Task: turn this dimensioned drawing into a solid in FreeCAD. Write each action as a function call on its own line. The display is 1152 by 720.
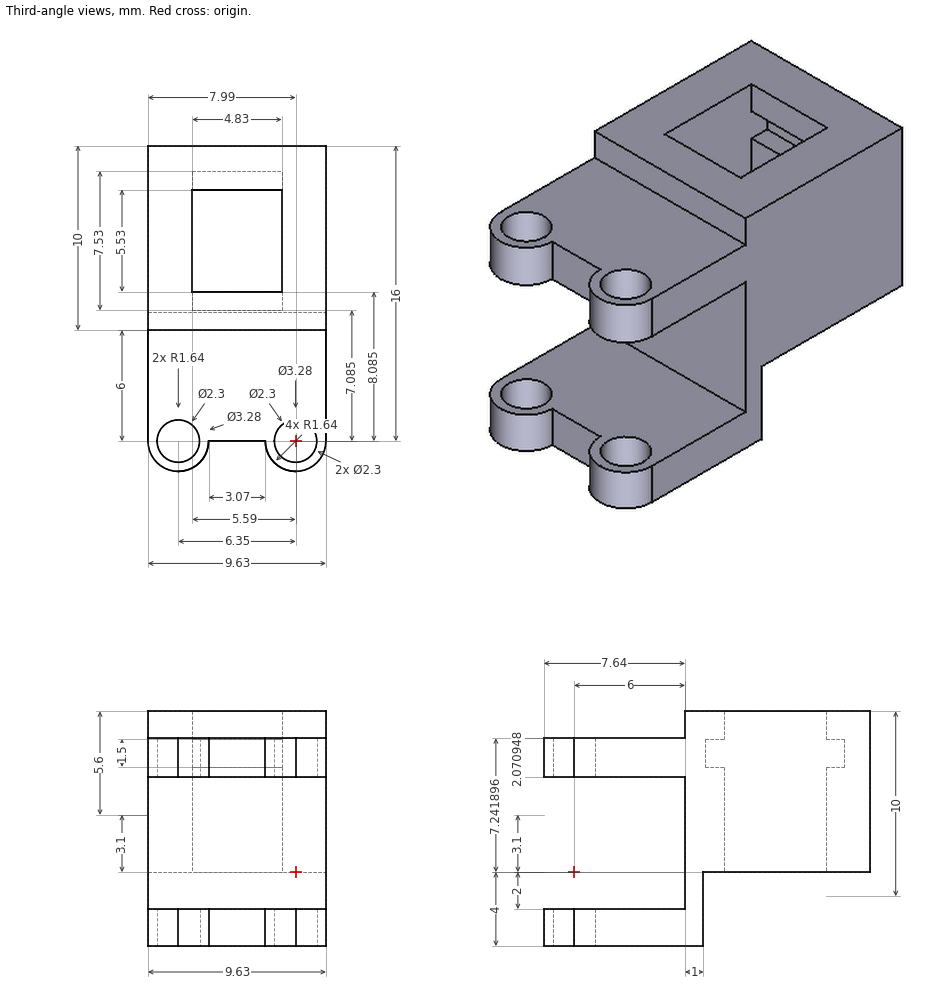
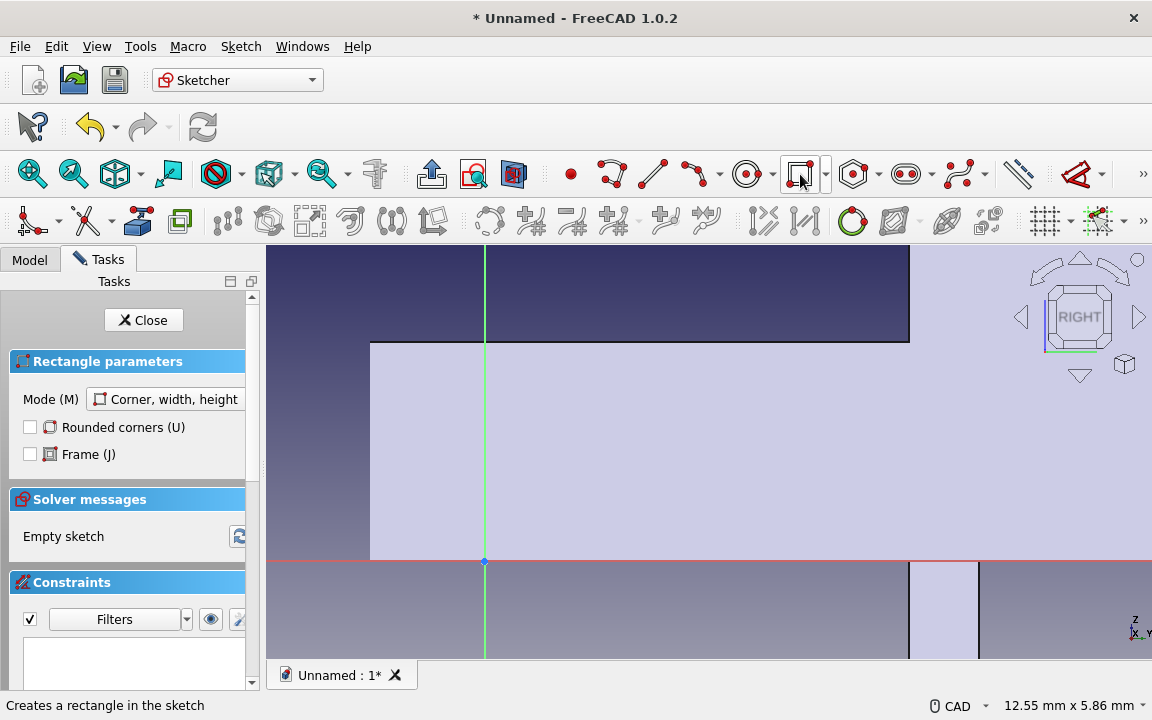
click(369, 342)
click(909, 561)
key(Escape)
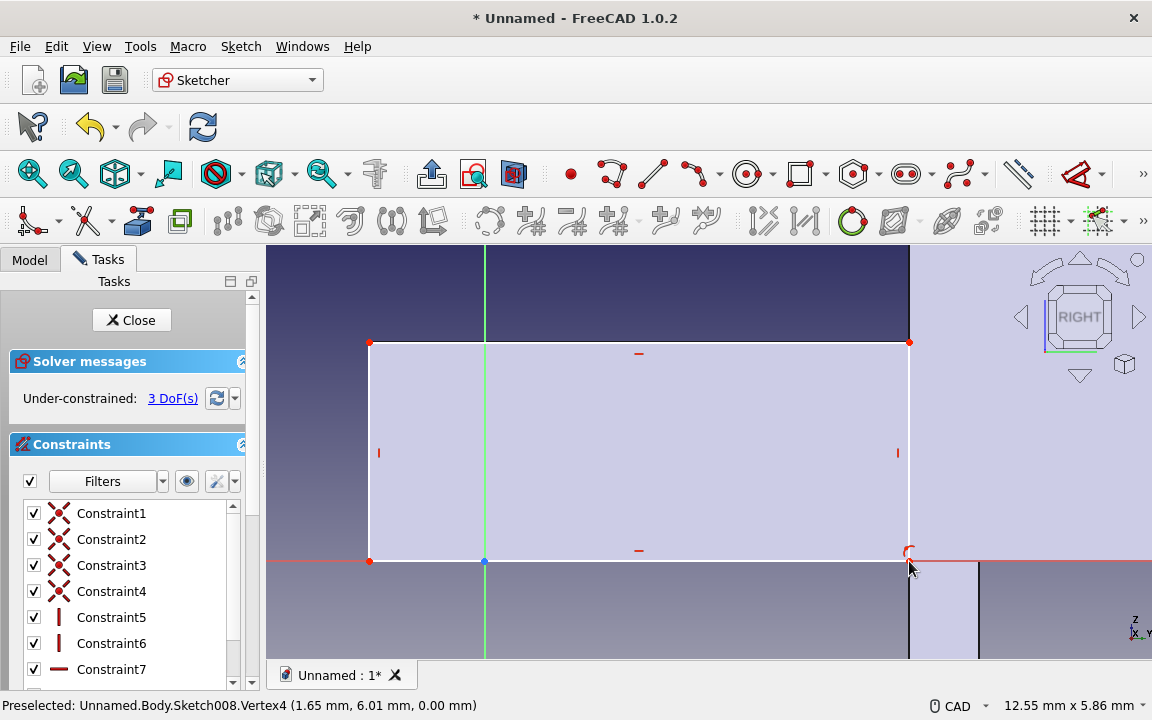
click(1076, 174)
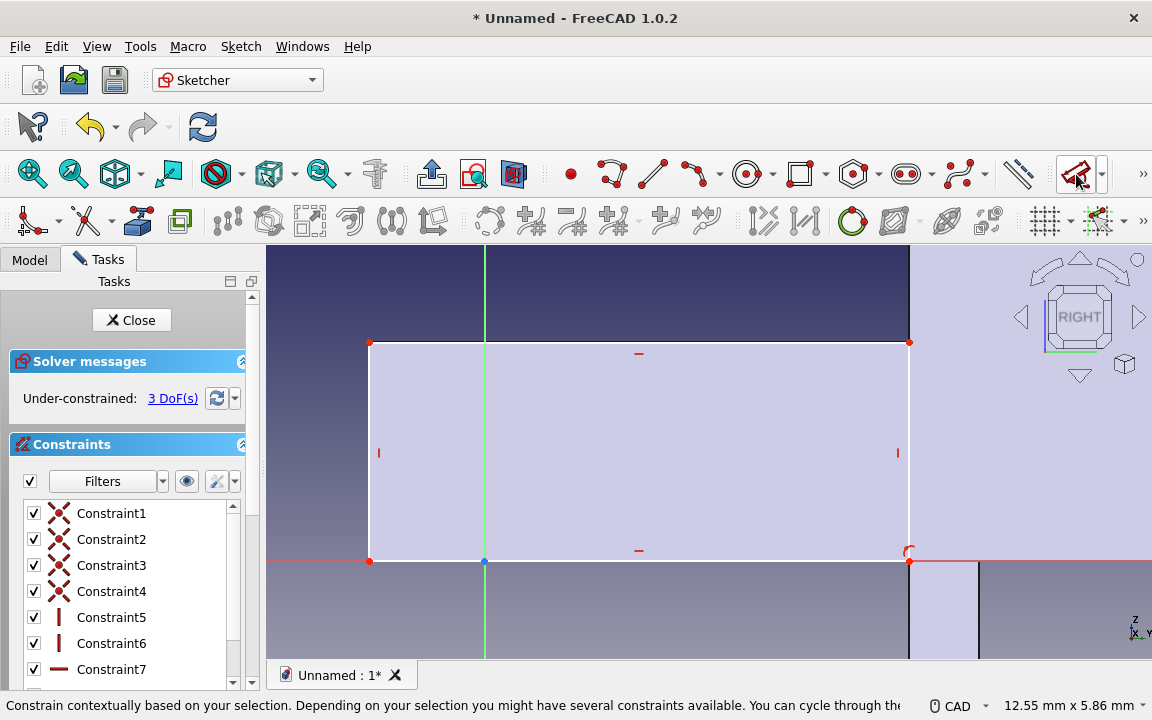
click(909, 561)
click(697, 595)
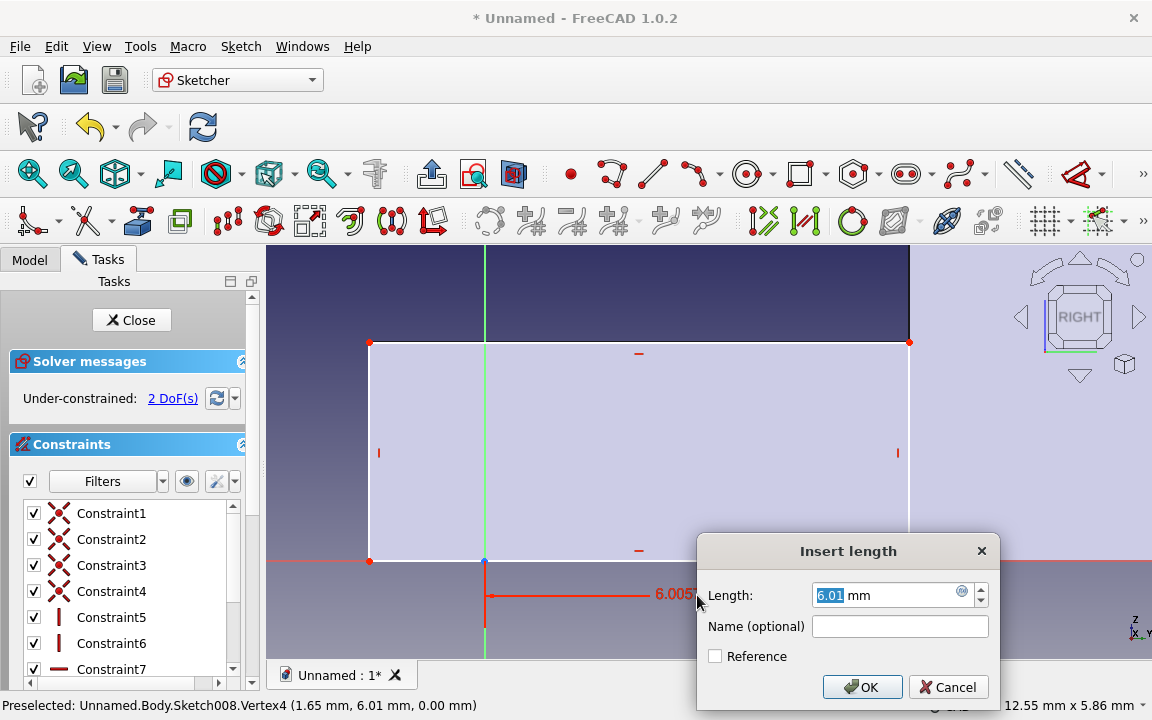
text(6)
key(Return)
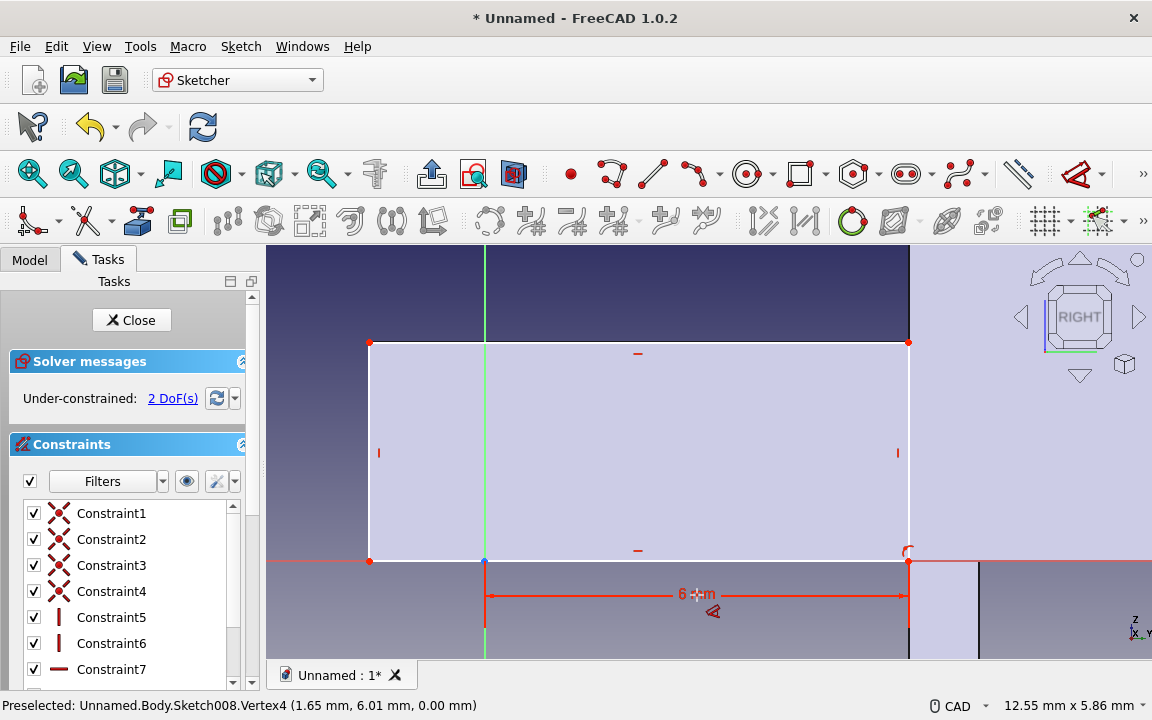
click(369, 408)
click(335, 452)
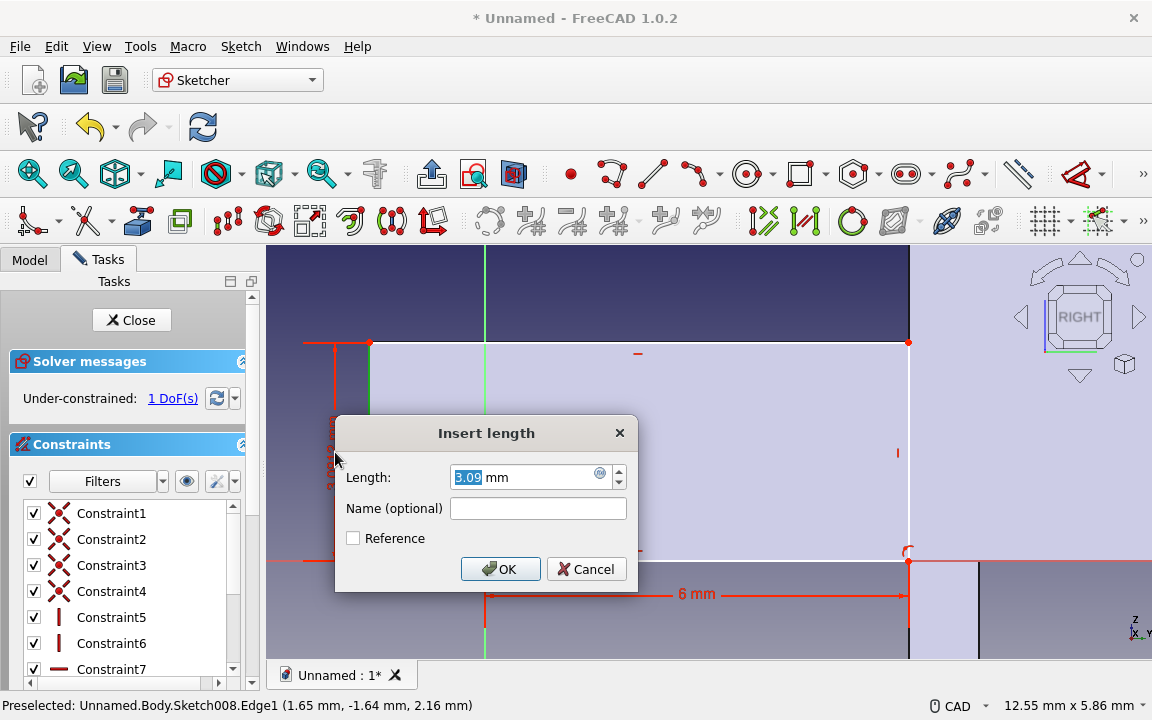
text(3.1)
key(Return)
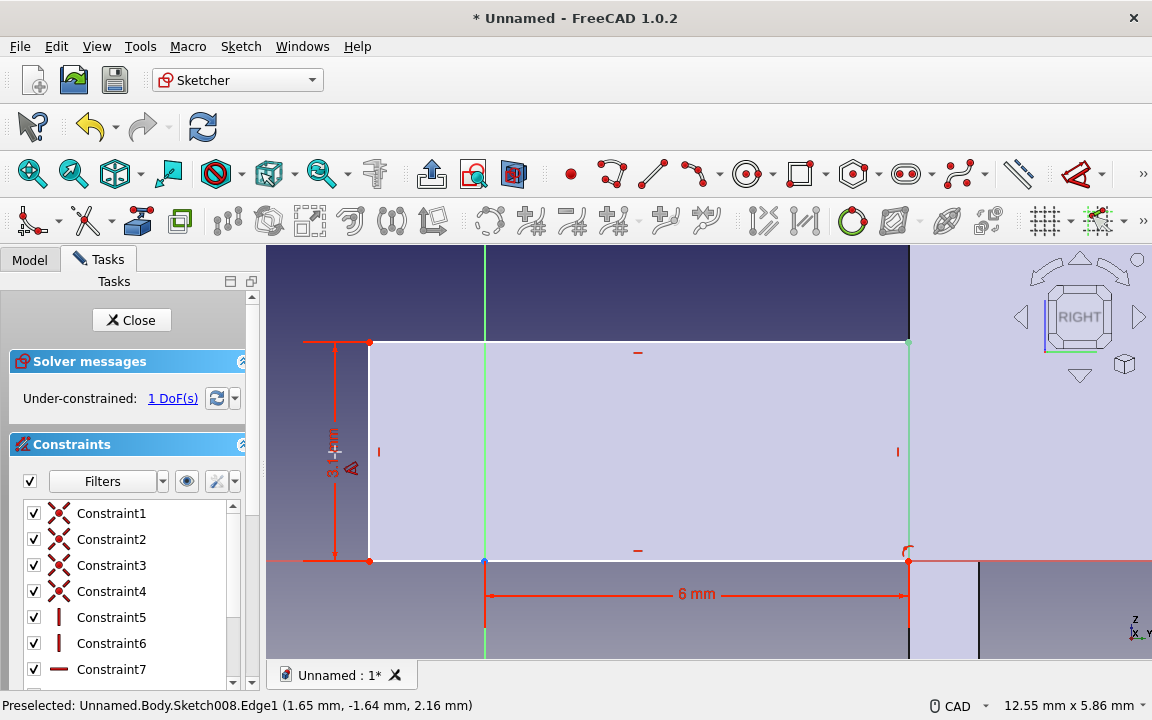
click(531, 561)
click(515, 595)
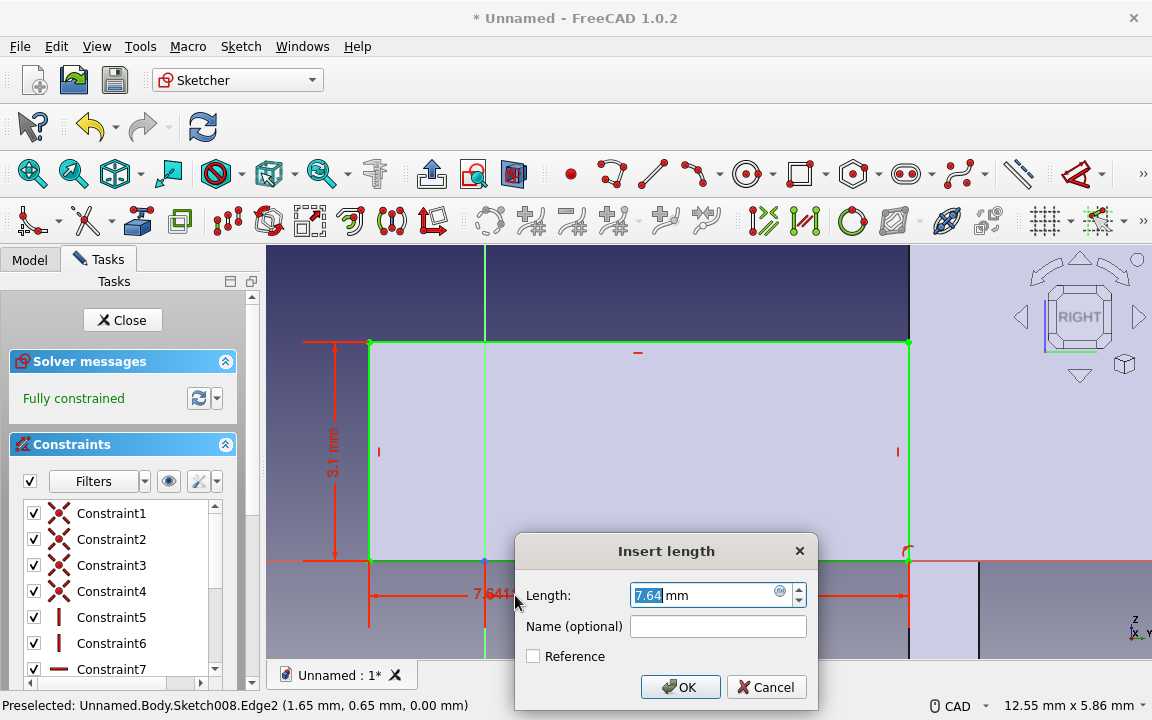
text(7.64)
key(Return)
key(Escape)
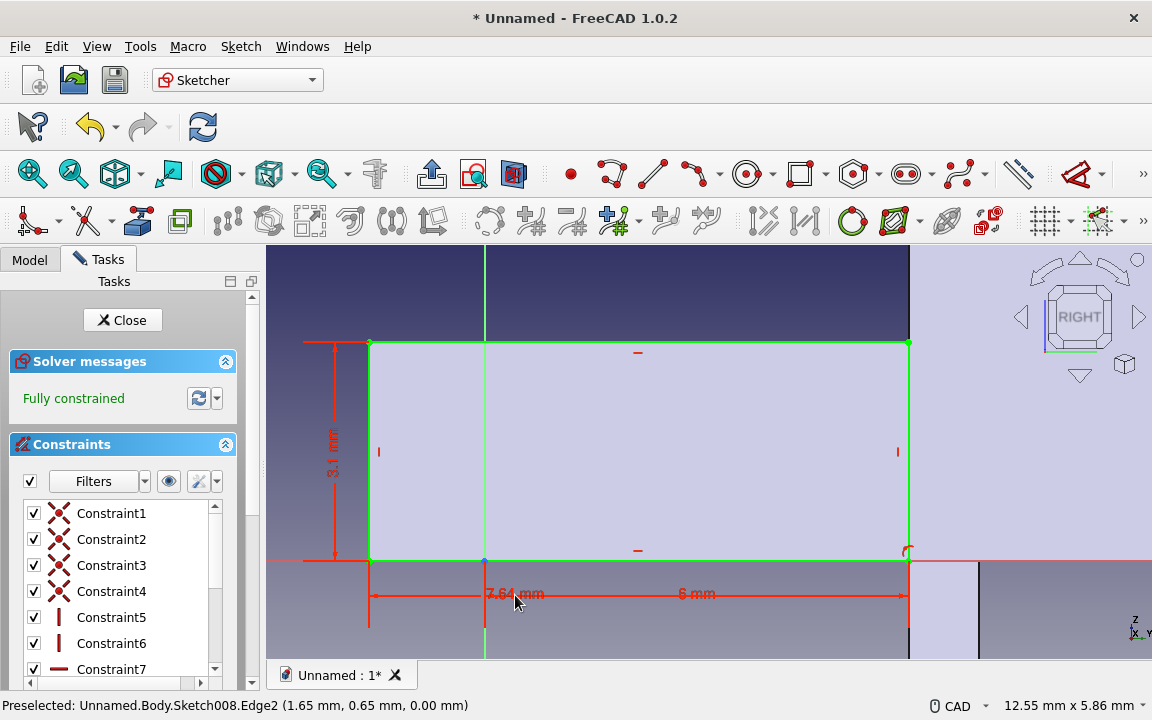
click(123, 320)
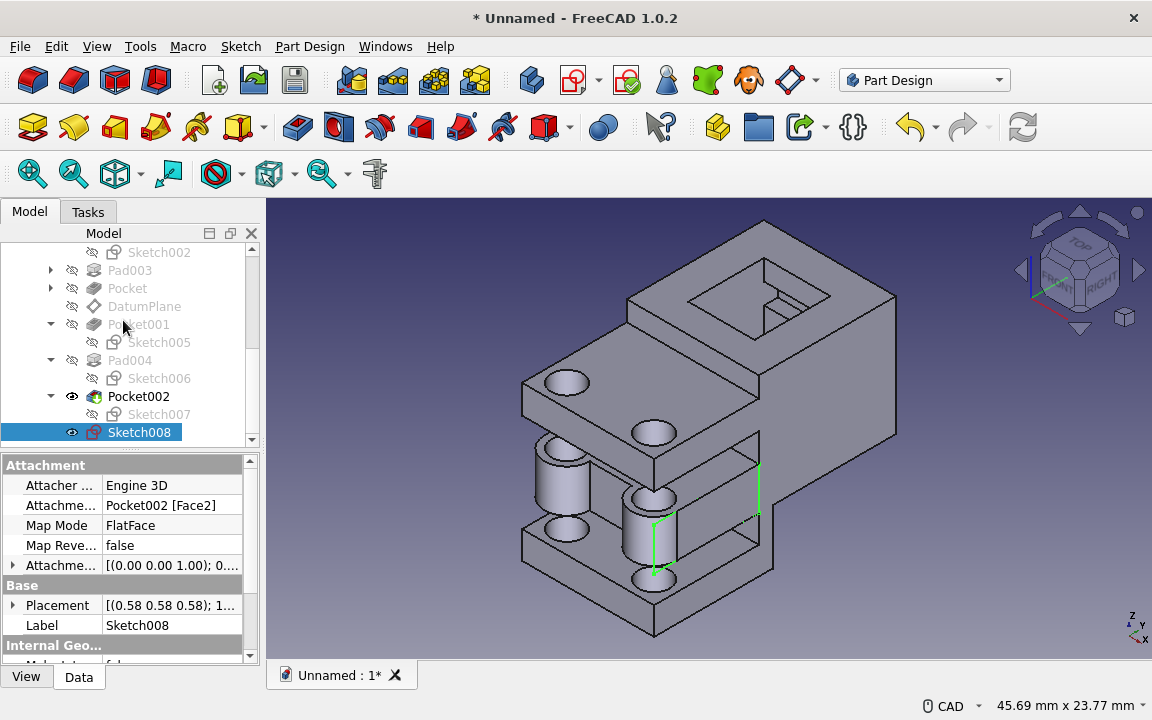
click(298, 128)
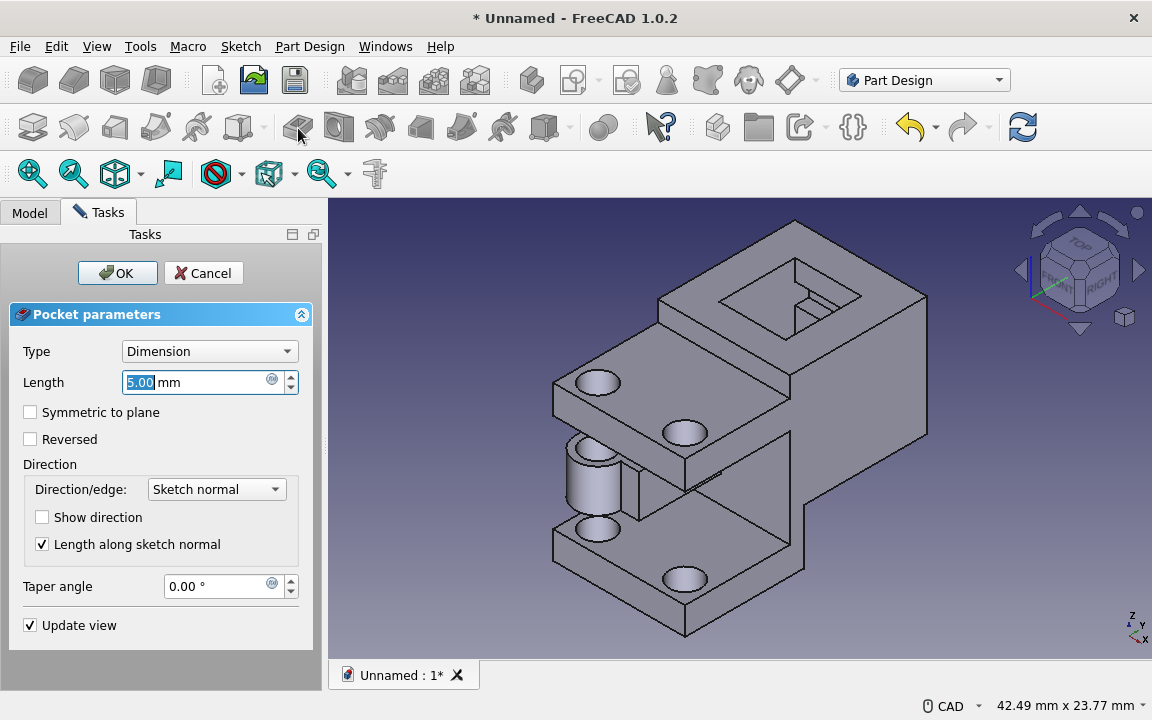
click(210, 352)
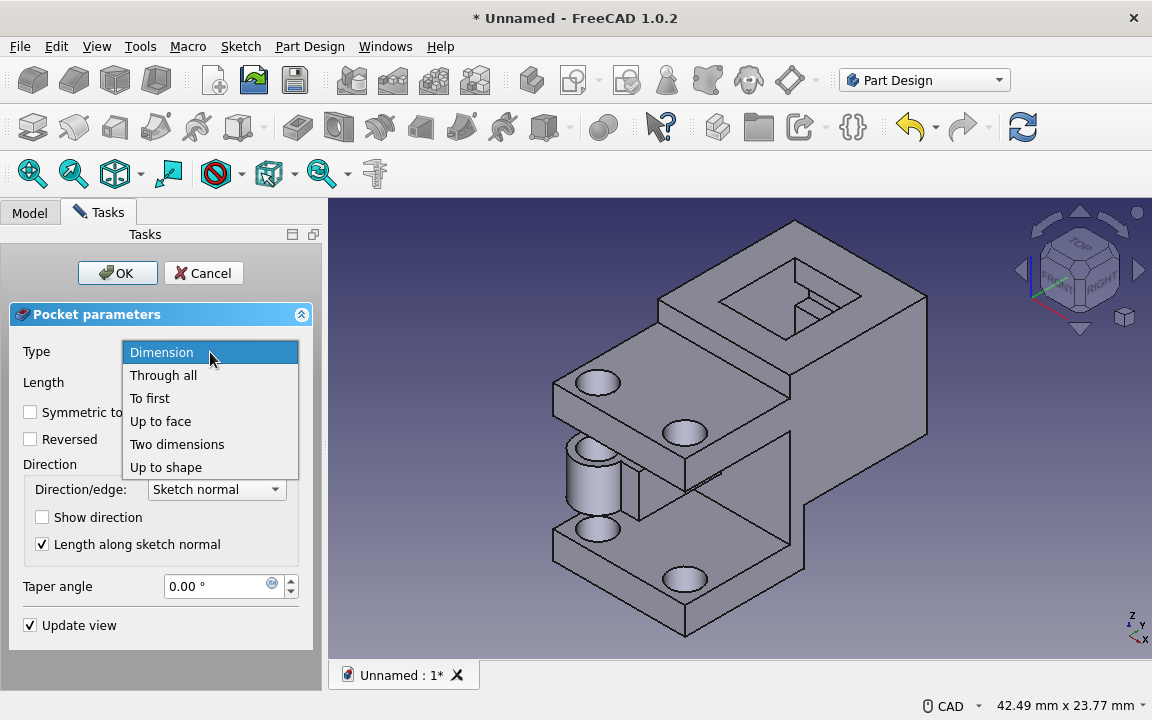
click(208, 376)